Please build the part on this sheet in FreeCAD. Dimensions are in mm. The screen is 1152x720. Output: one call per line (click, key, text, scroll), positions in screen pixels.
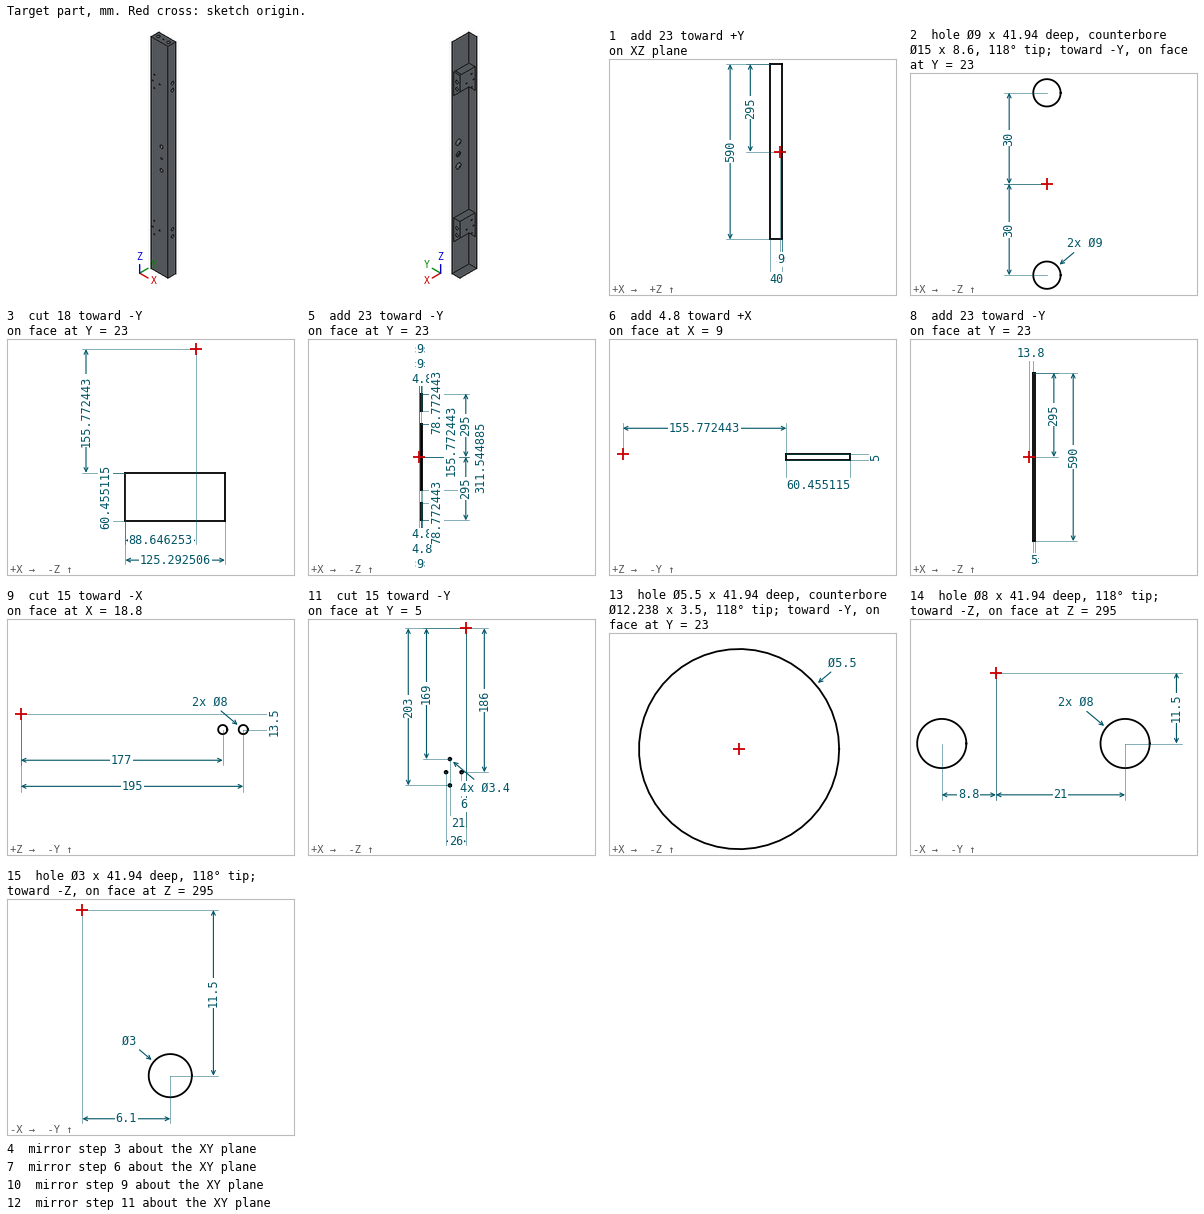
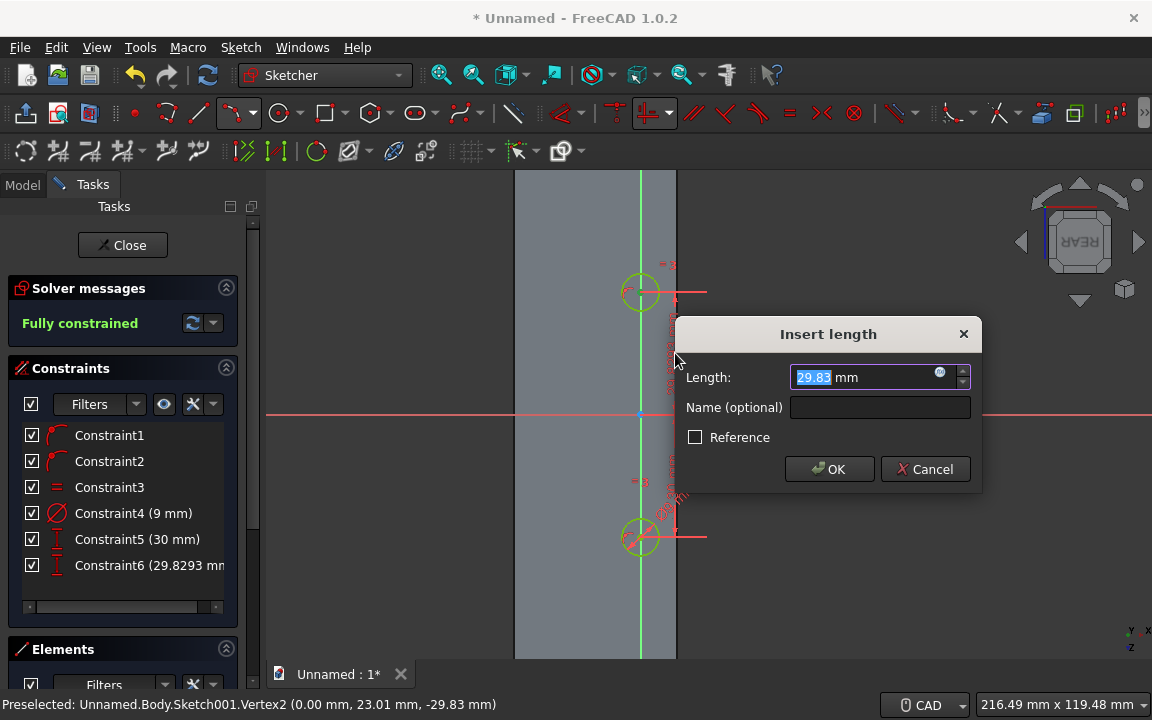
text(30)
key(Return)
key(Escape)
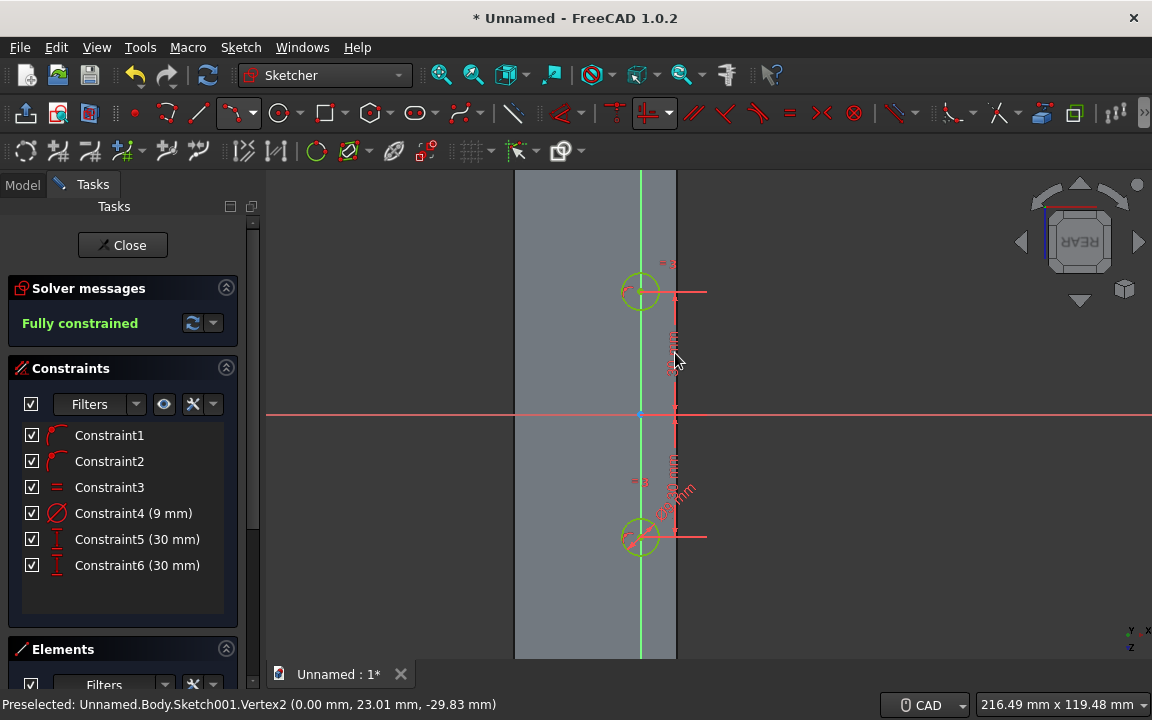
click(123, 245)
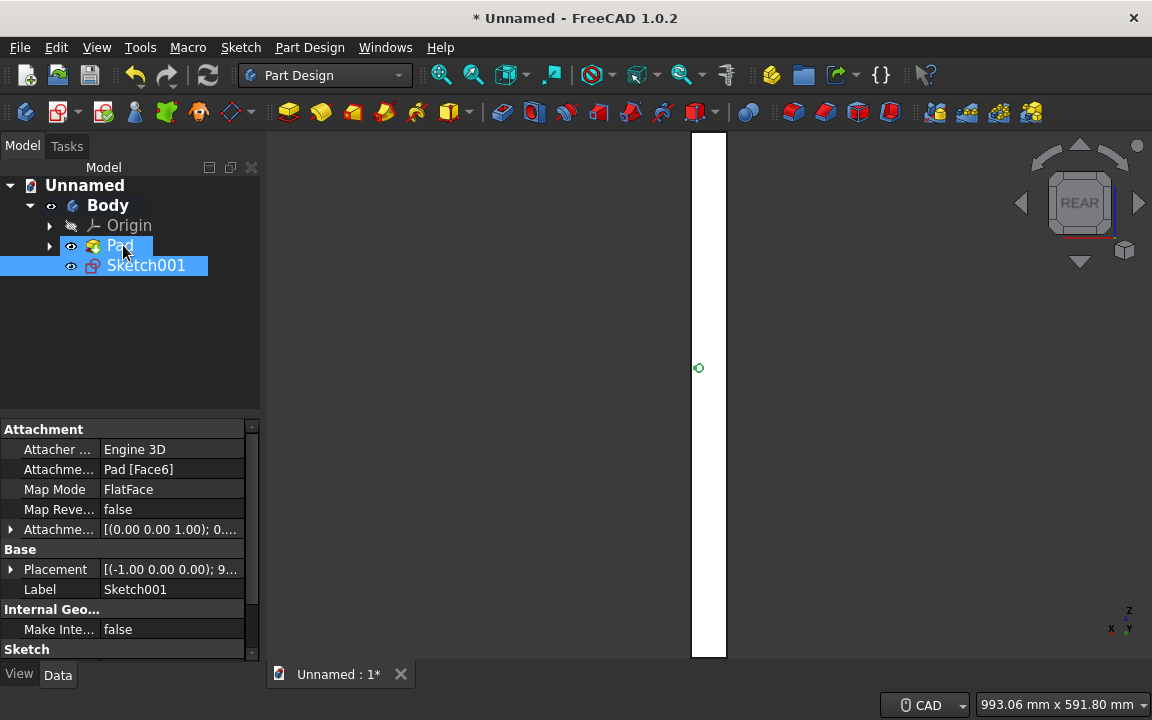
click(536, 112)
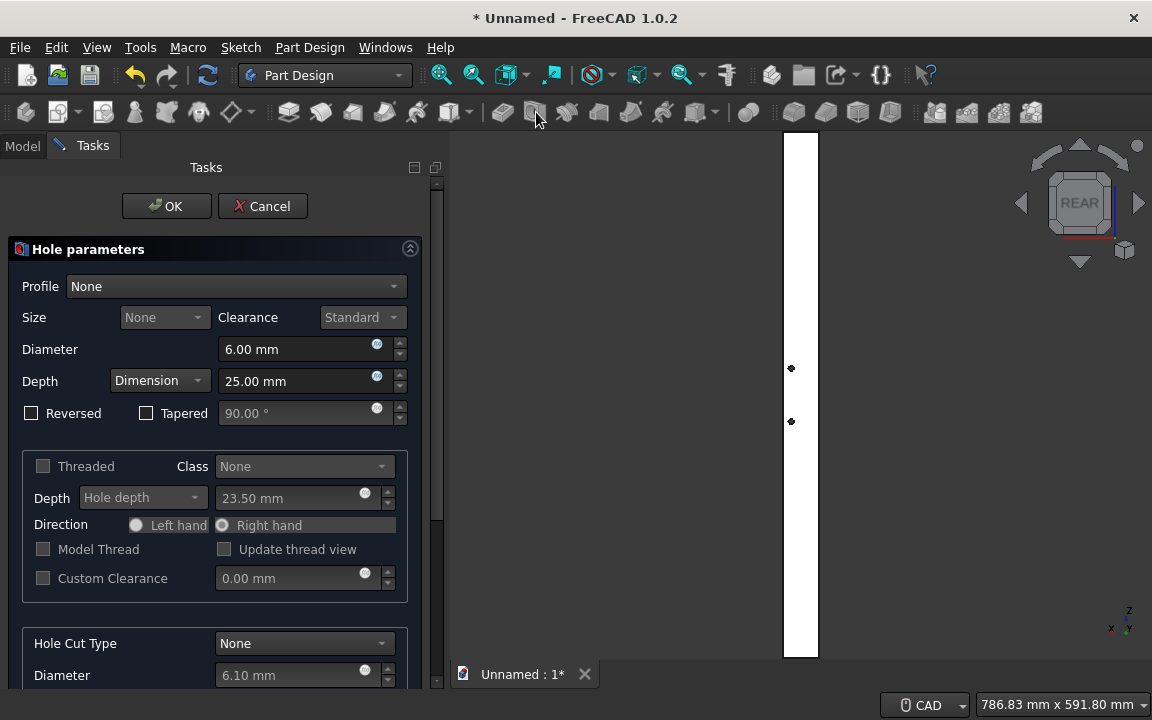
triple_click(305, 349)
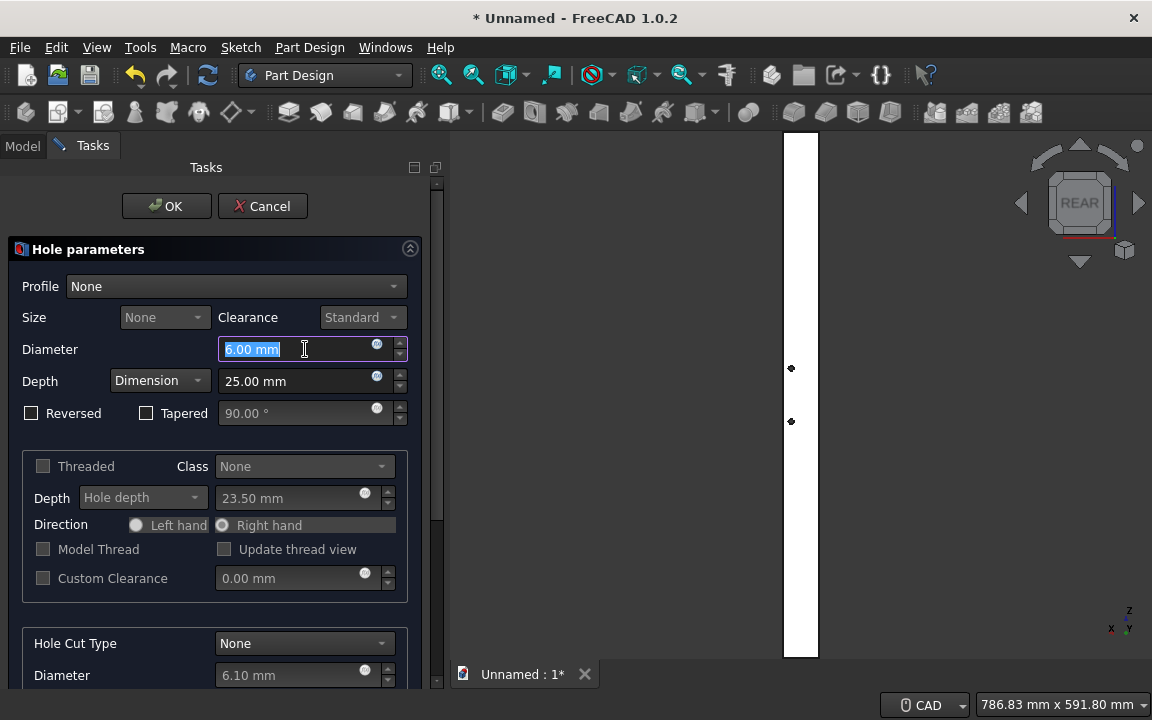
text(9)
key(Tab)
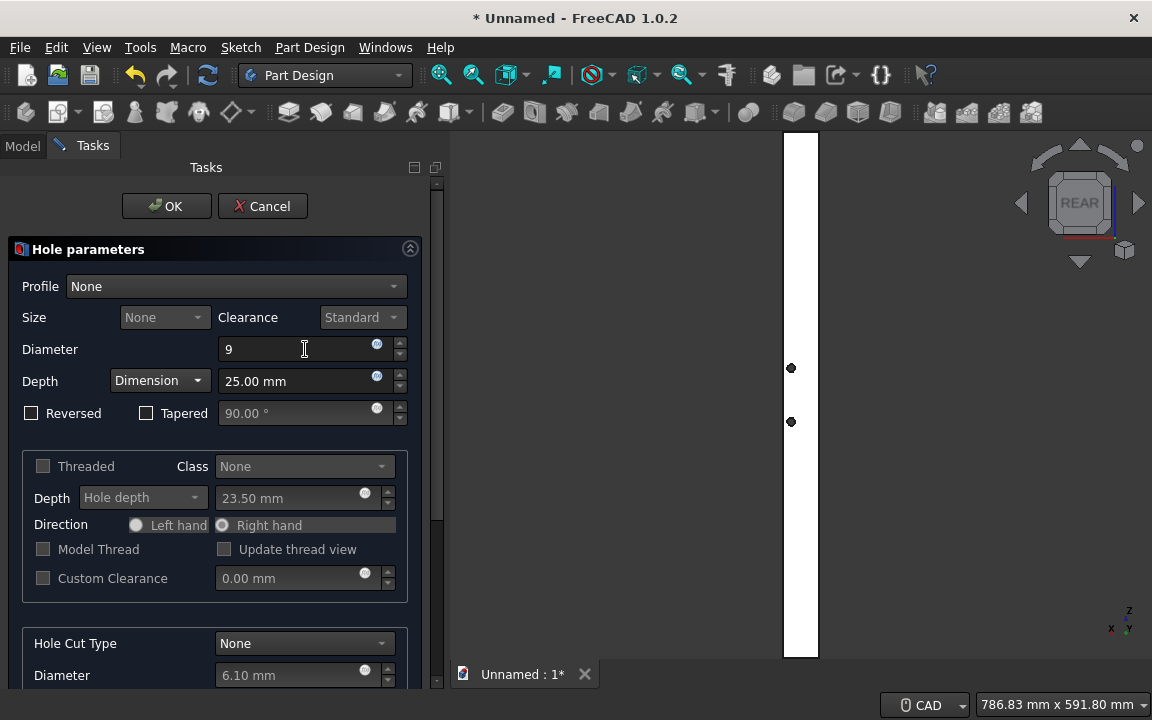
triple_click(305, 381)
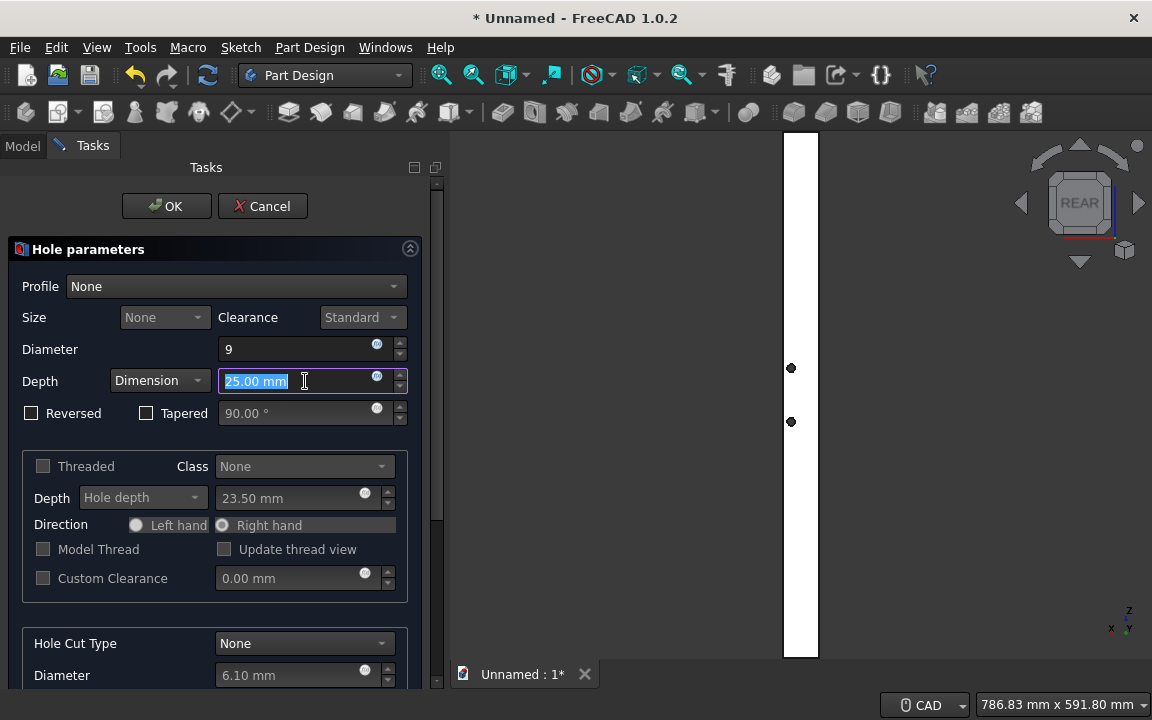
text(41.94)
key(Tab)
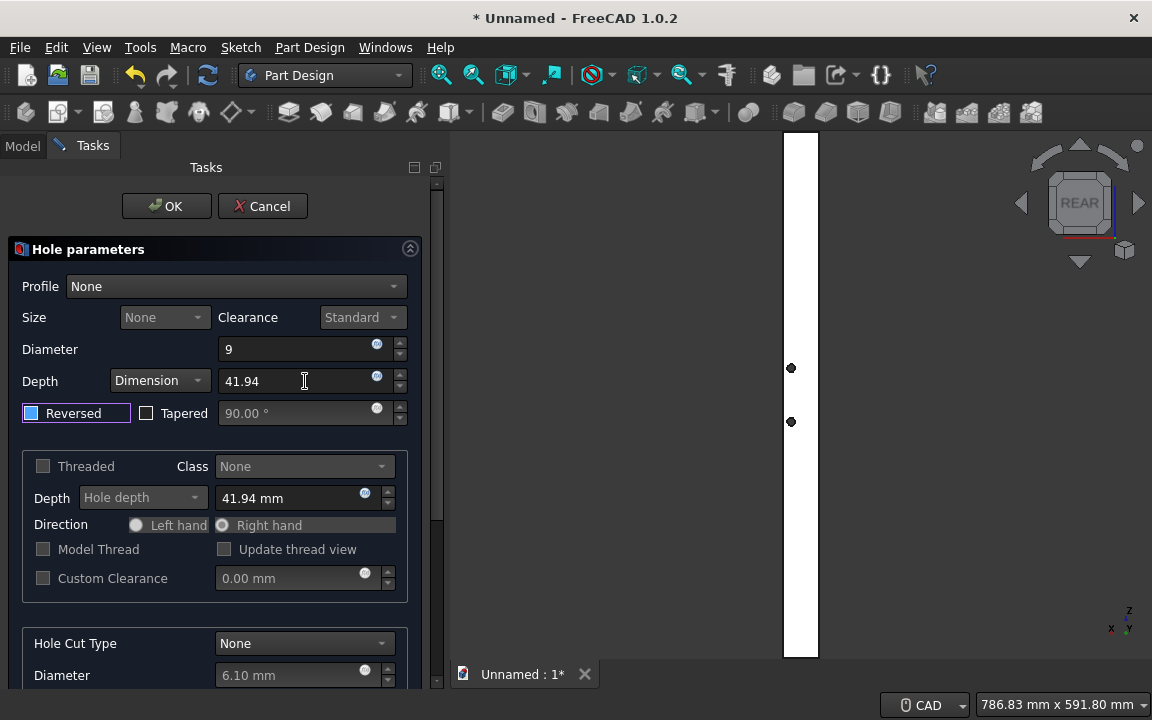
click(306, 644)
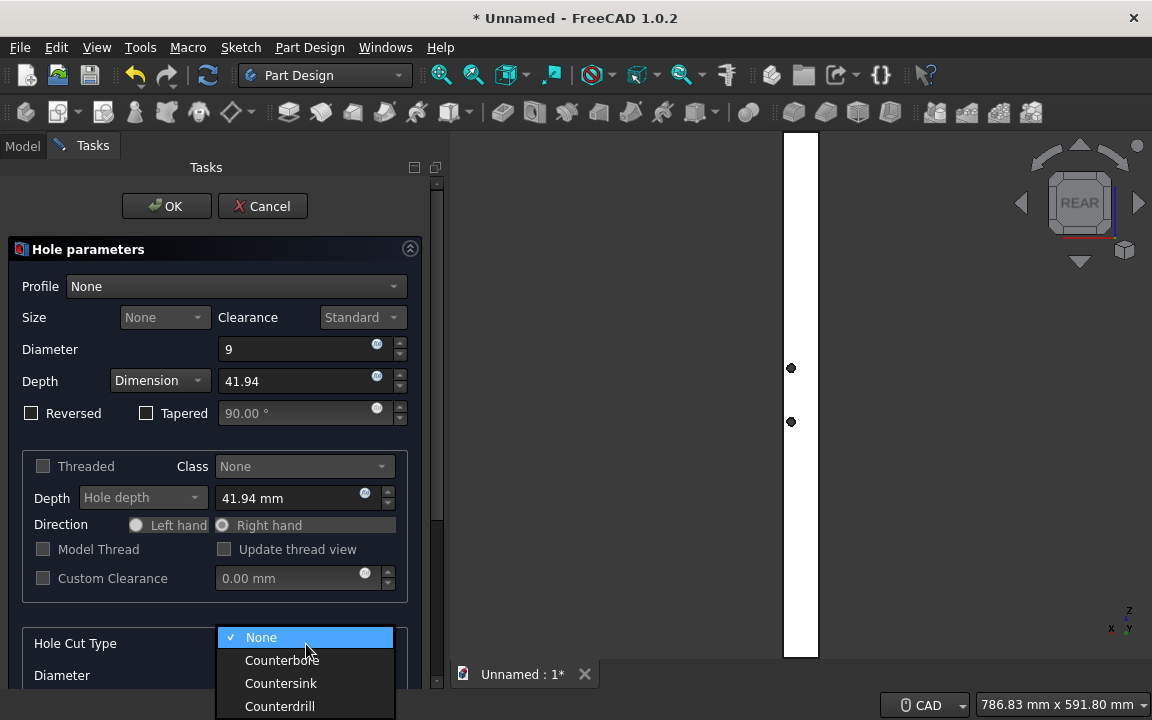
click(304, 660)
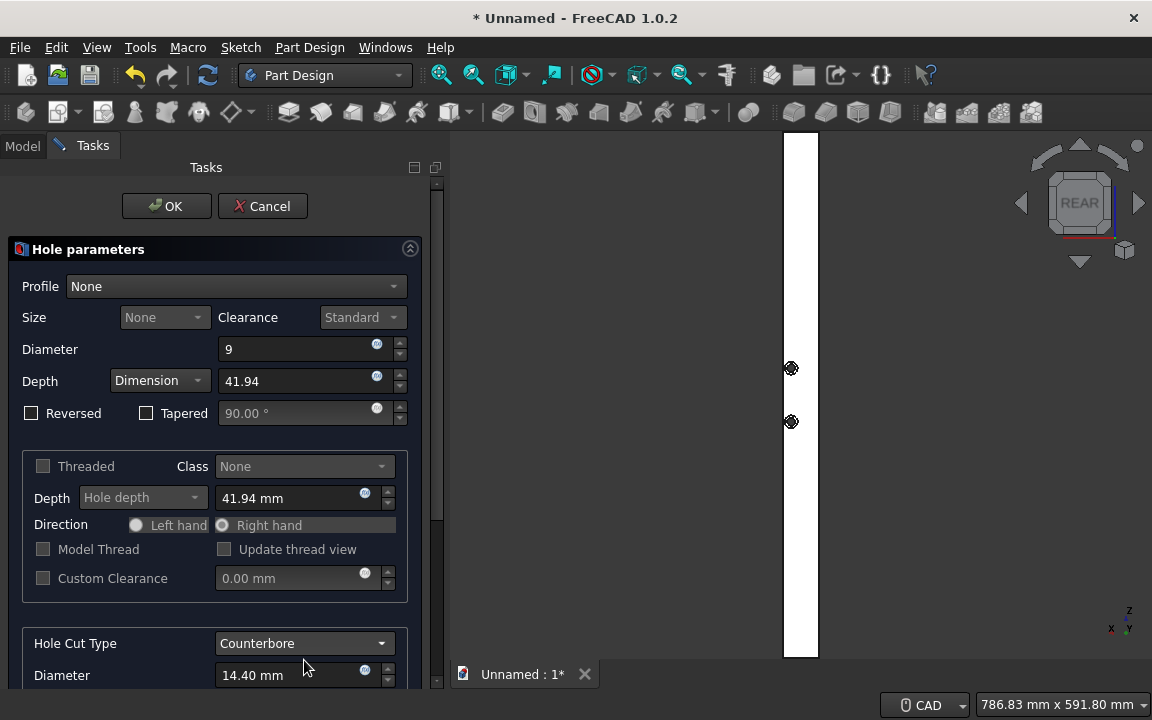
triple_click(298, 675)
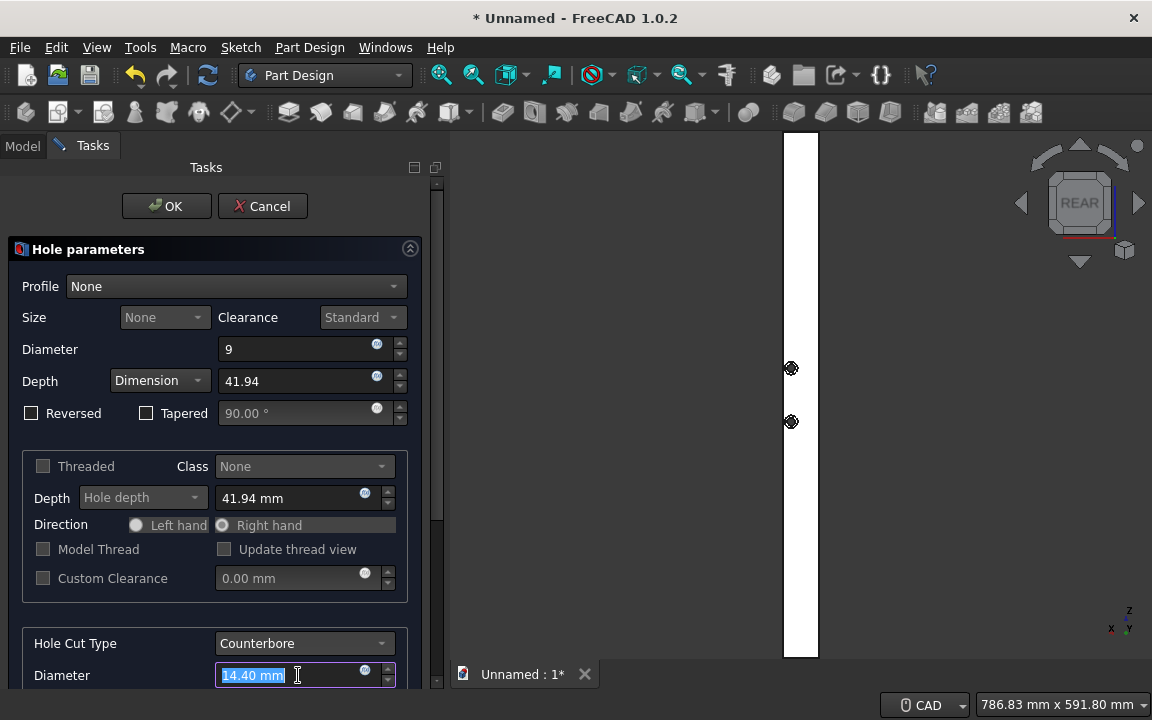
text(15)
key(Tab)